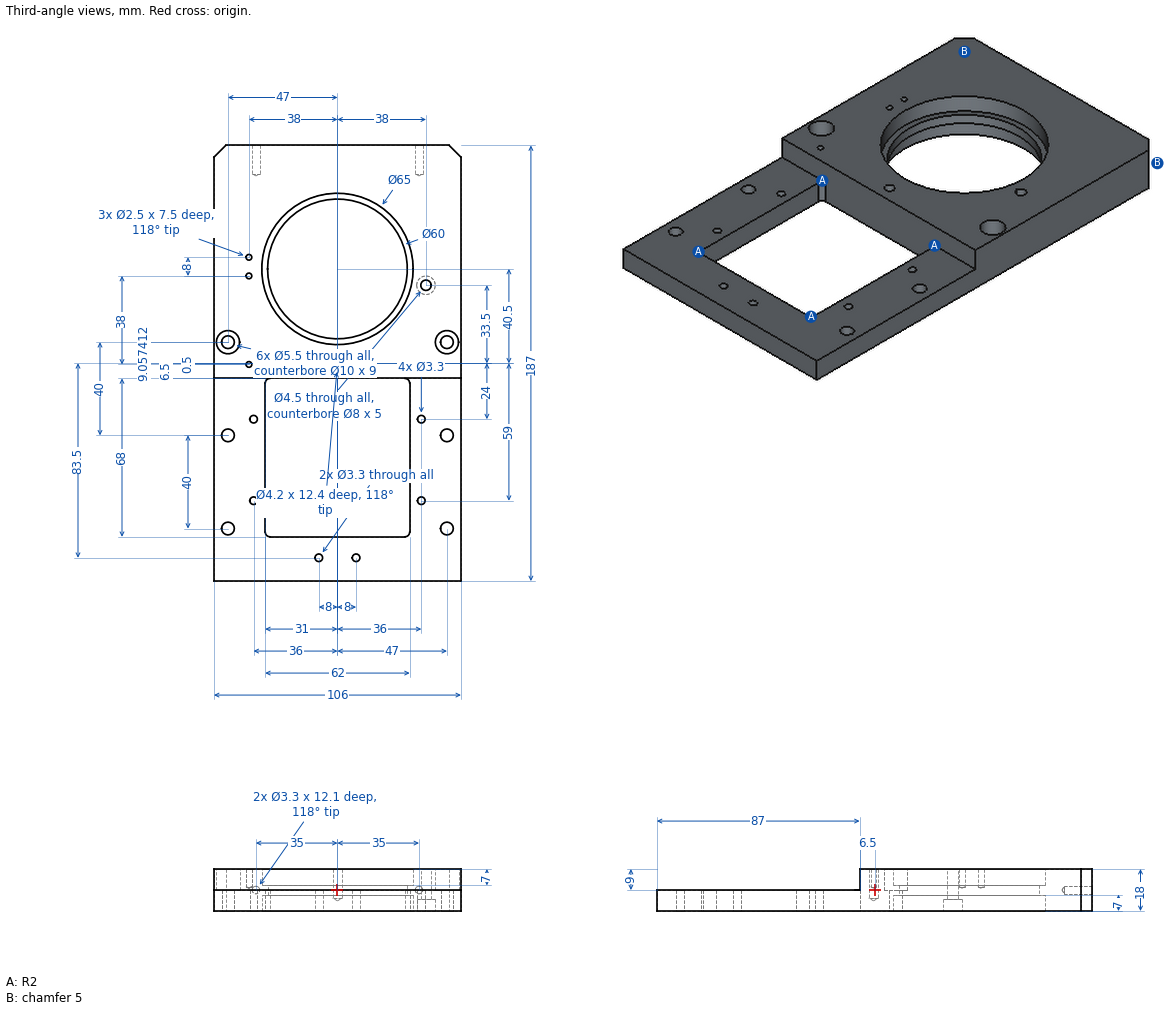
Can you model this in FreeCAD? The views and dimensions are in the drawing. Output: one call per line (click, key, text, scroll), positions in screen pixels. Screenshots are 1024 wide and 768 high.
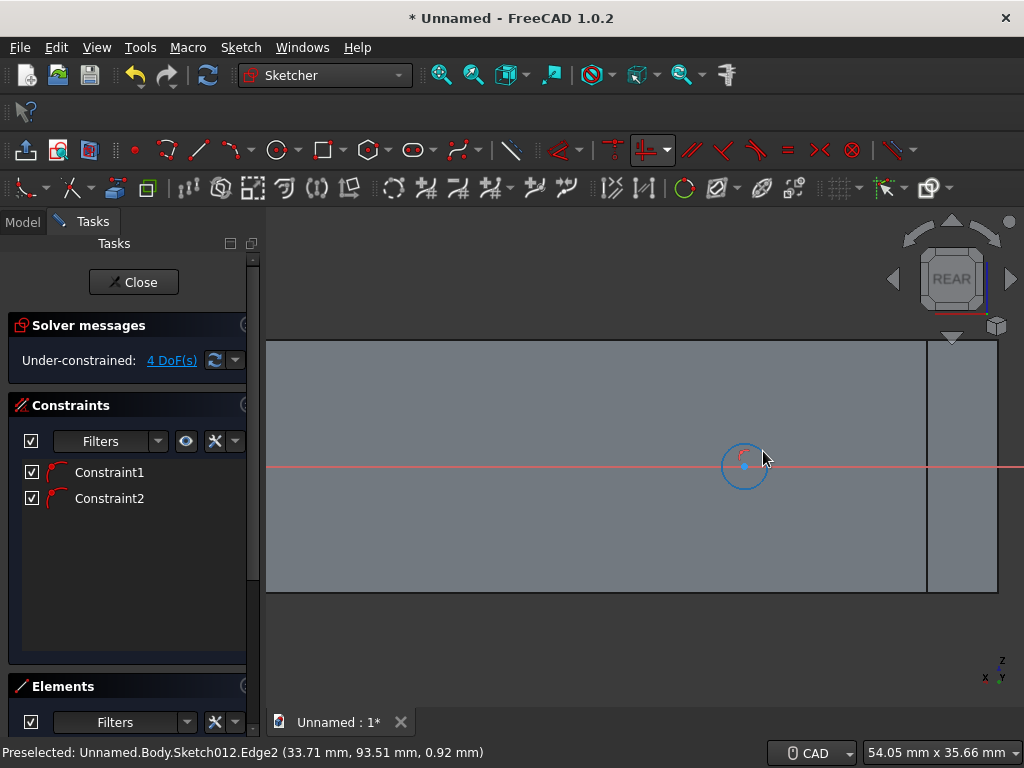
click(761, 450)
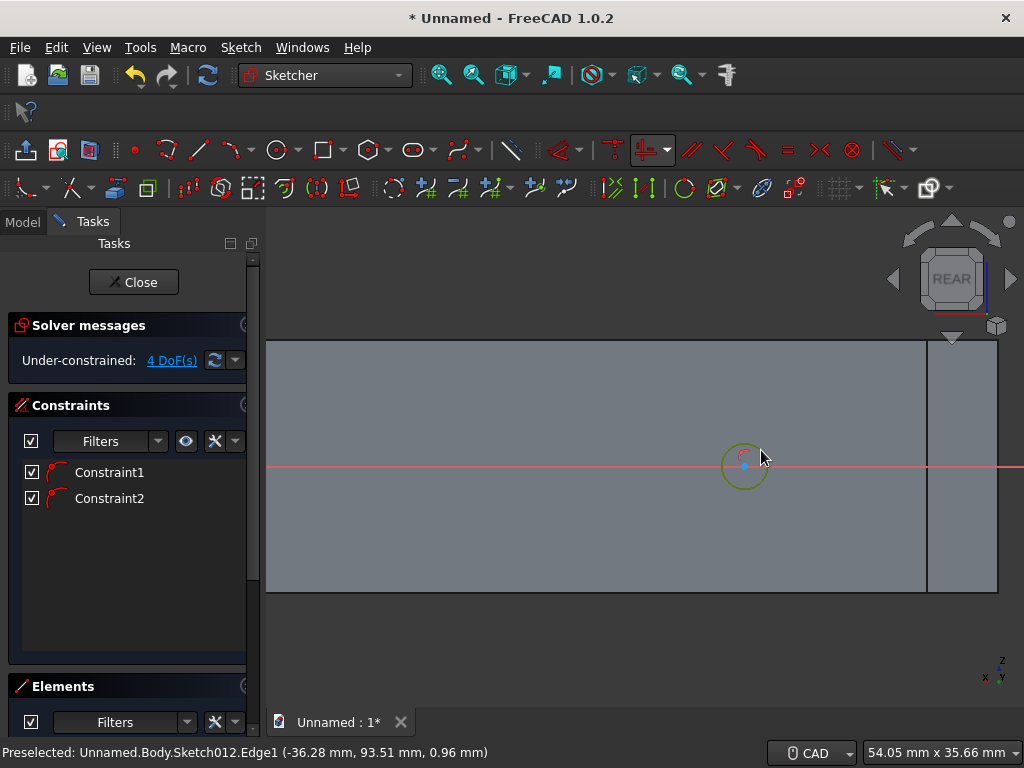
scroll(764, 451, down, 5)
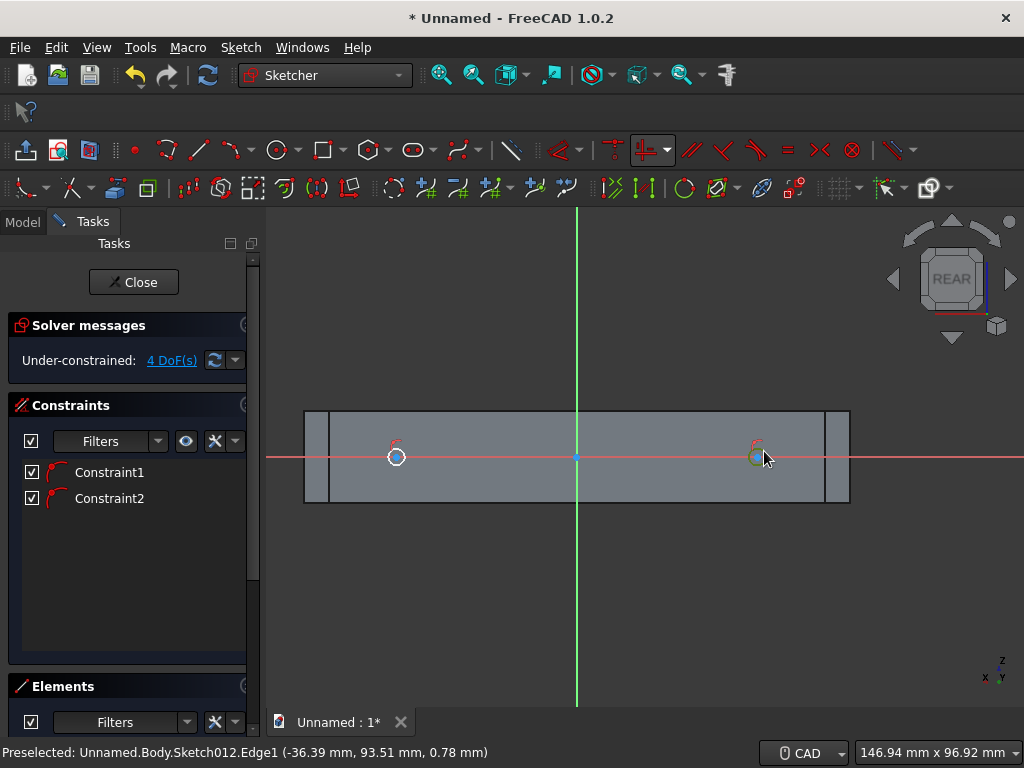
scroll(402, 451, up, 5)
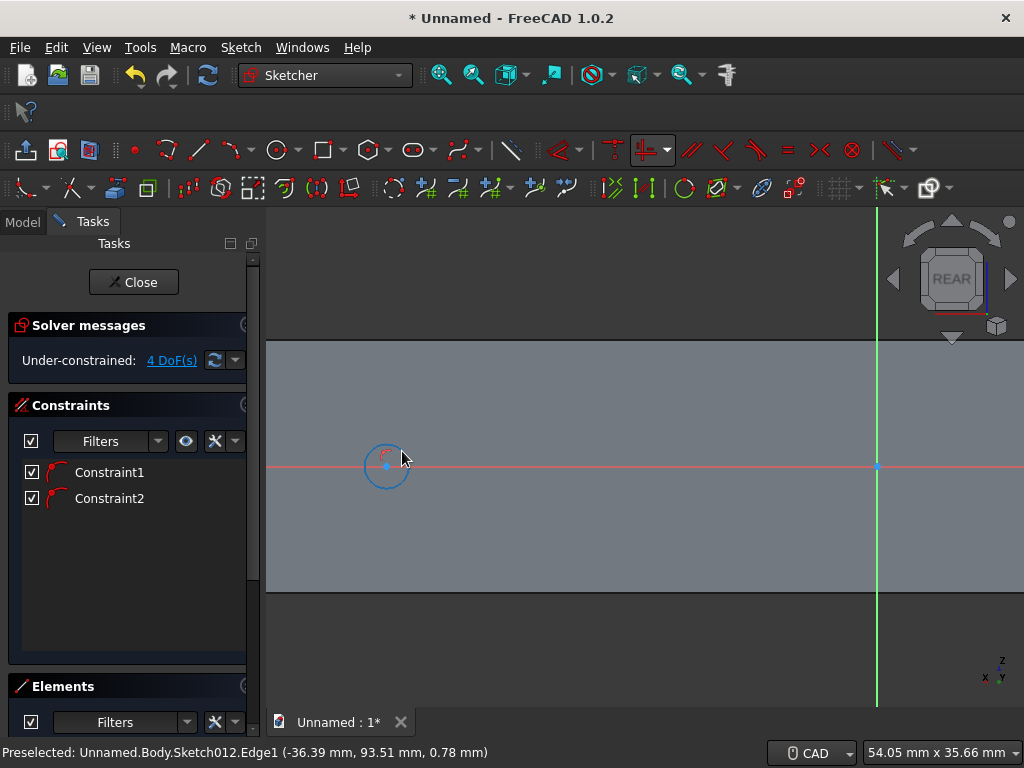
click(402, 451)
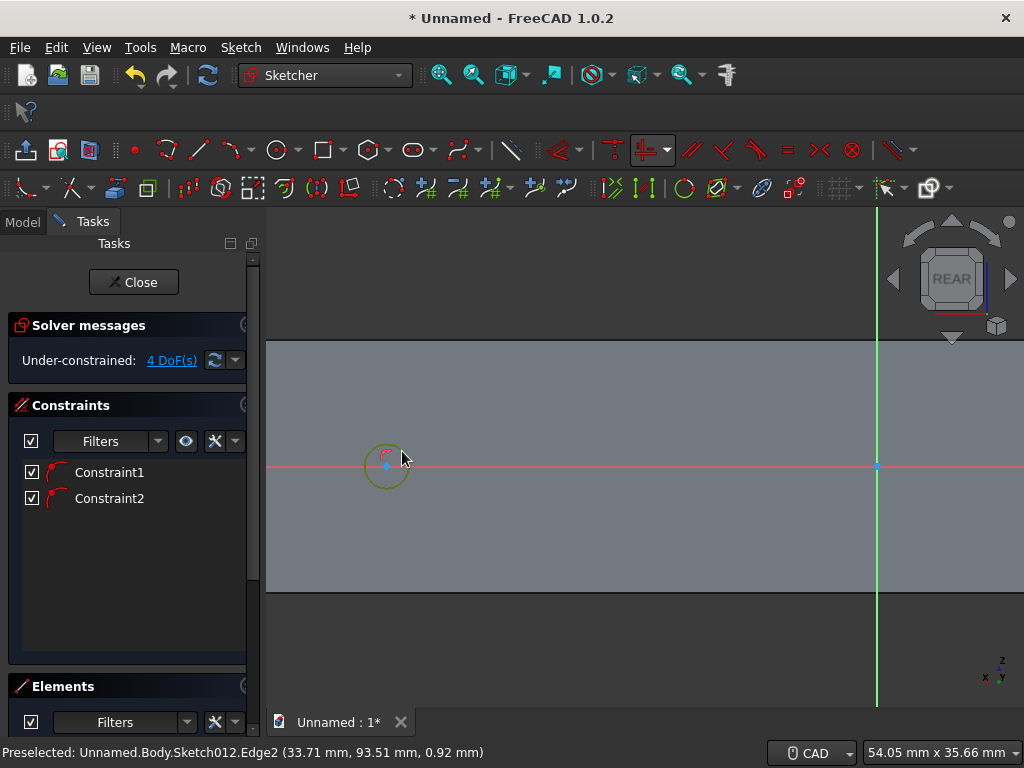
click(788, 150)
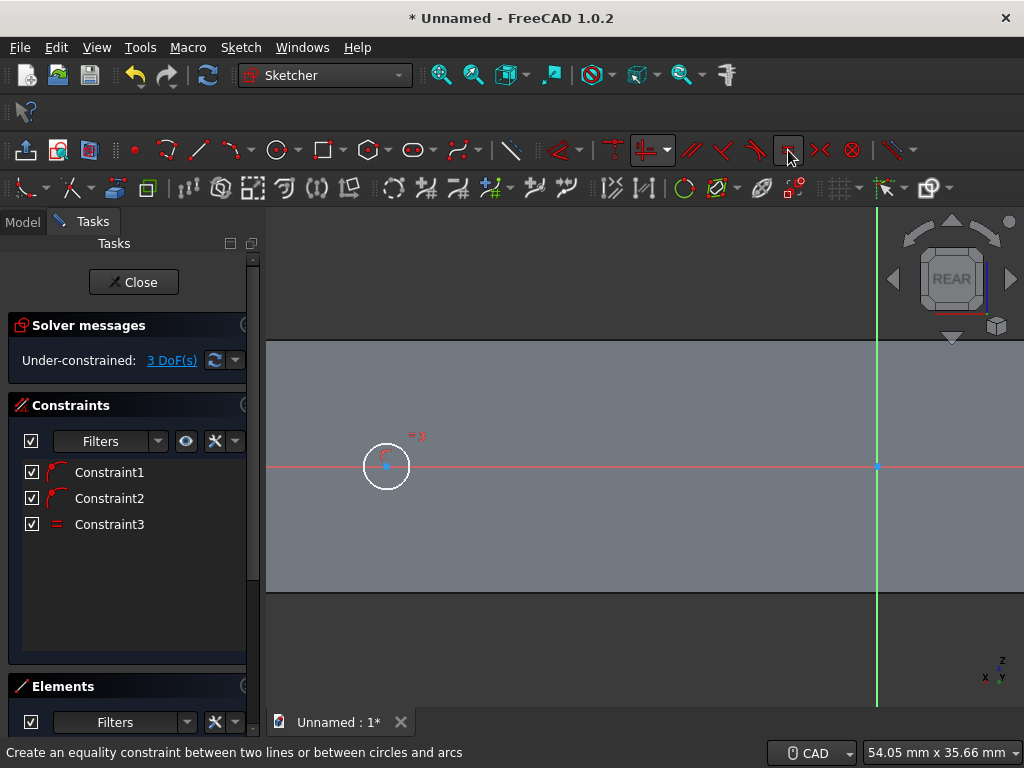
click(558, 150)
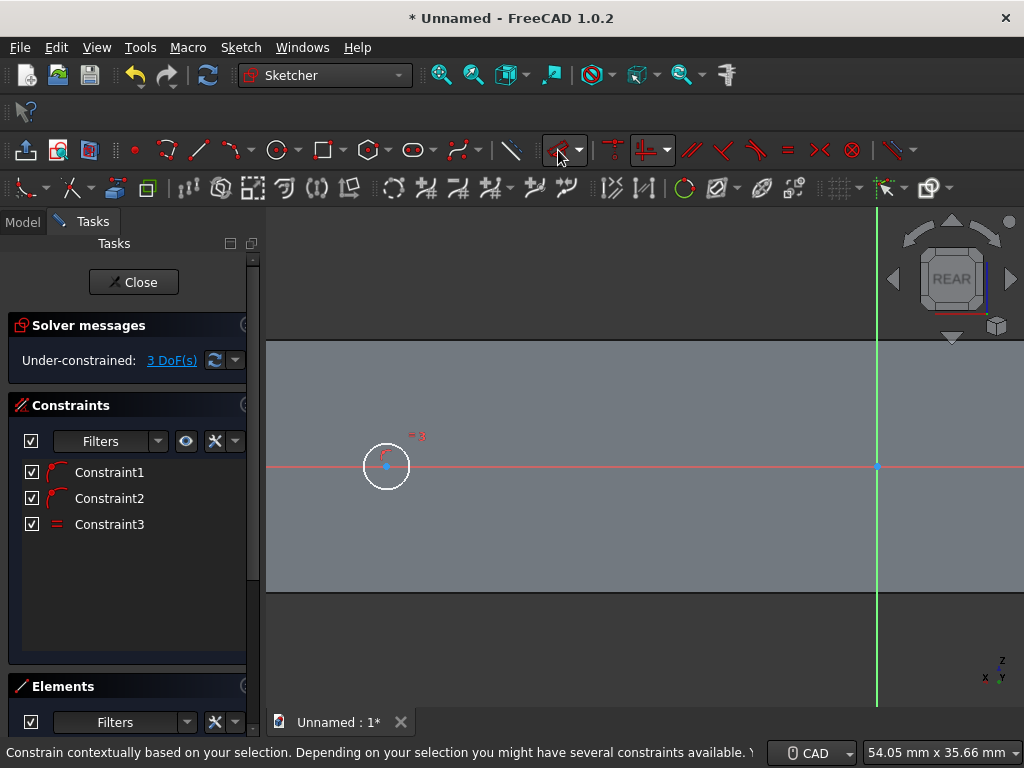
scroll(401, 451, down, 5)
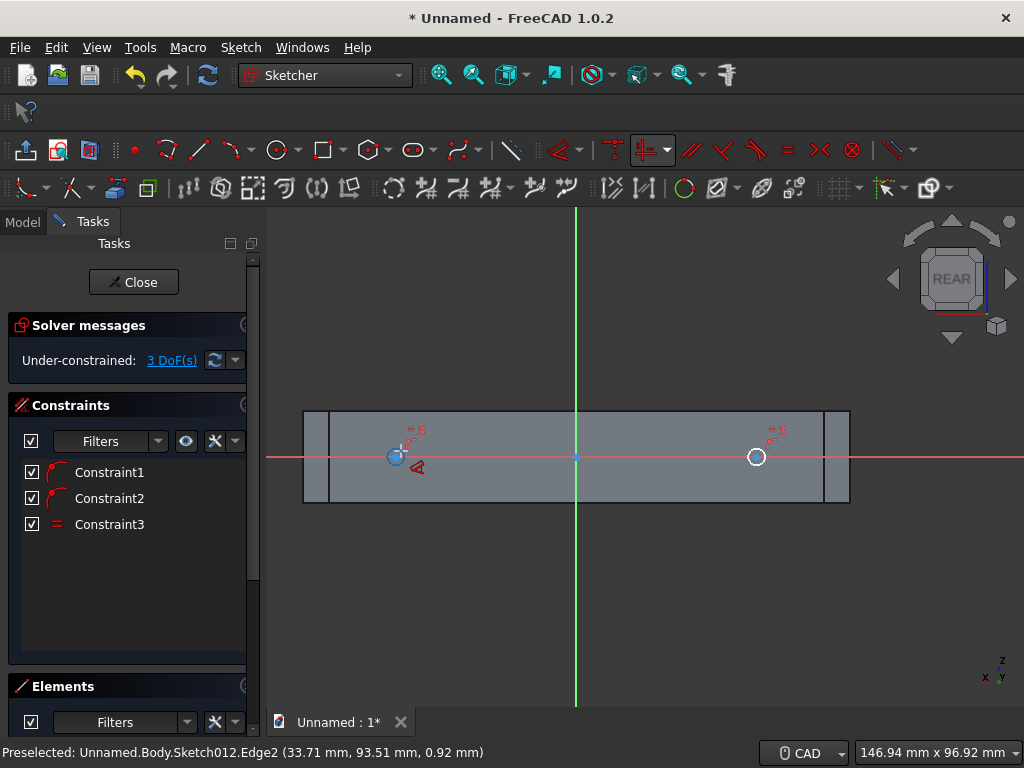
scroll(763, 451, up, 5)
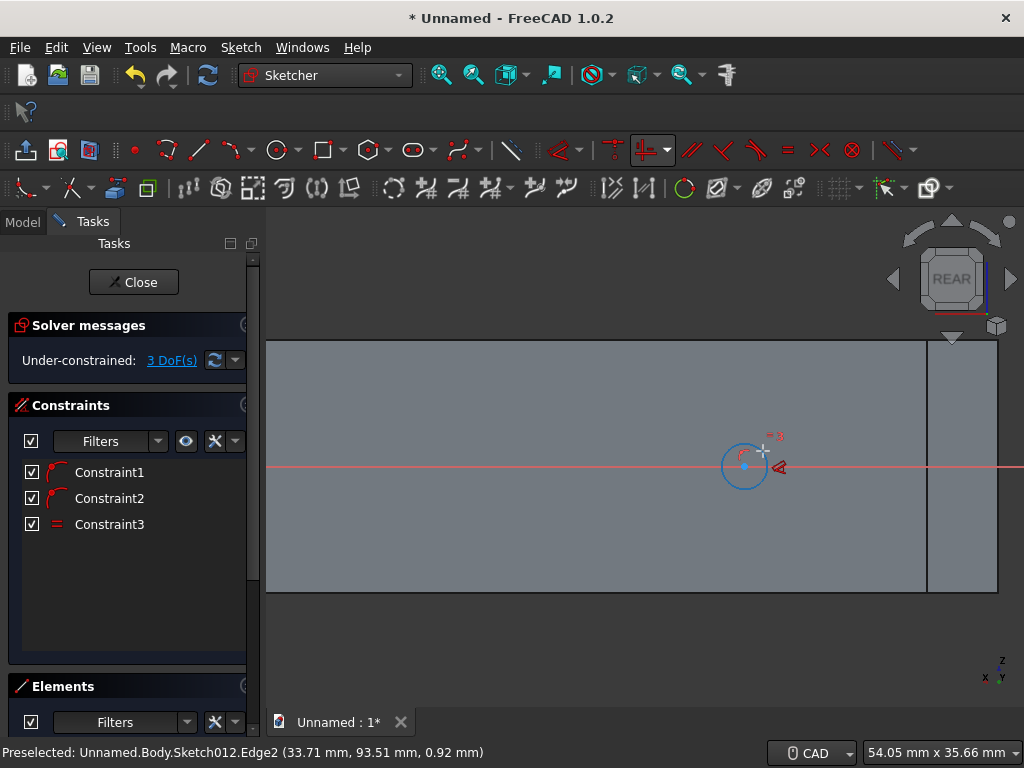
click(761, 450)
click(783, 427)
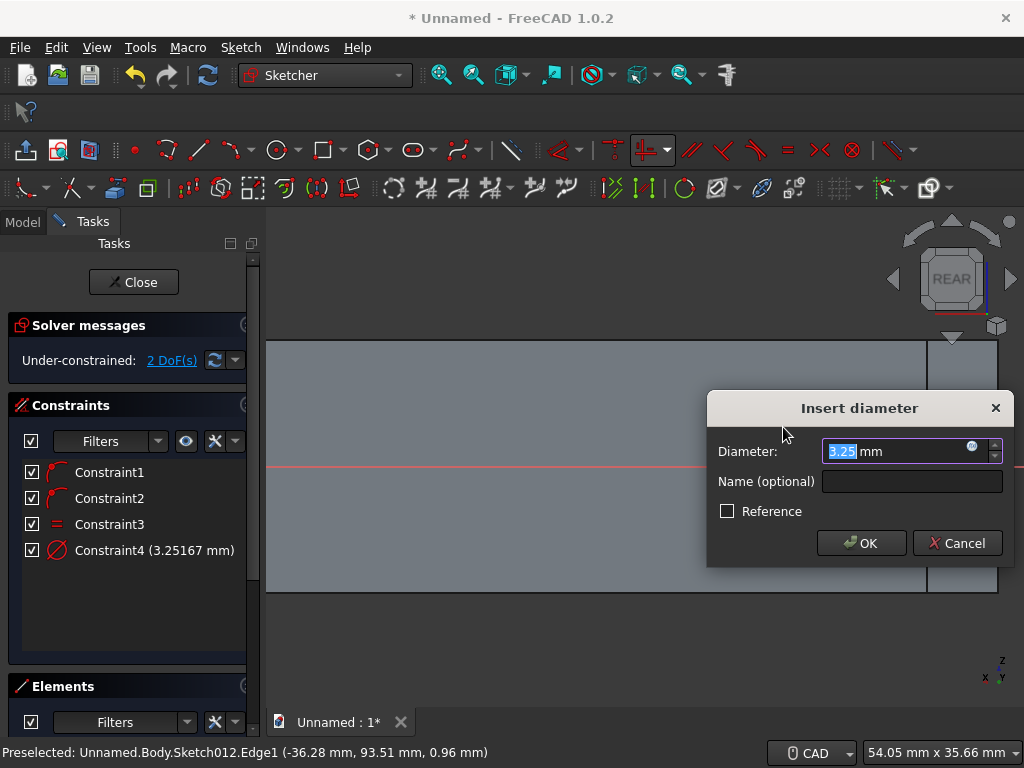
text(3.3)
key(Return)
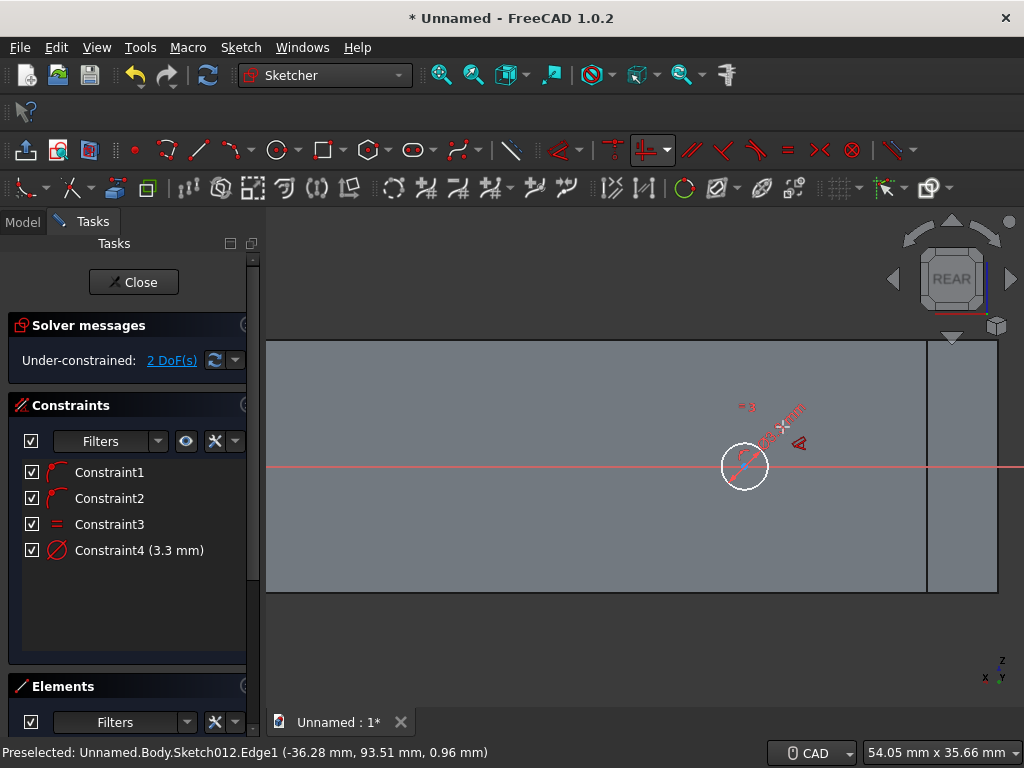
click(745, 467)
click(519, 501)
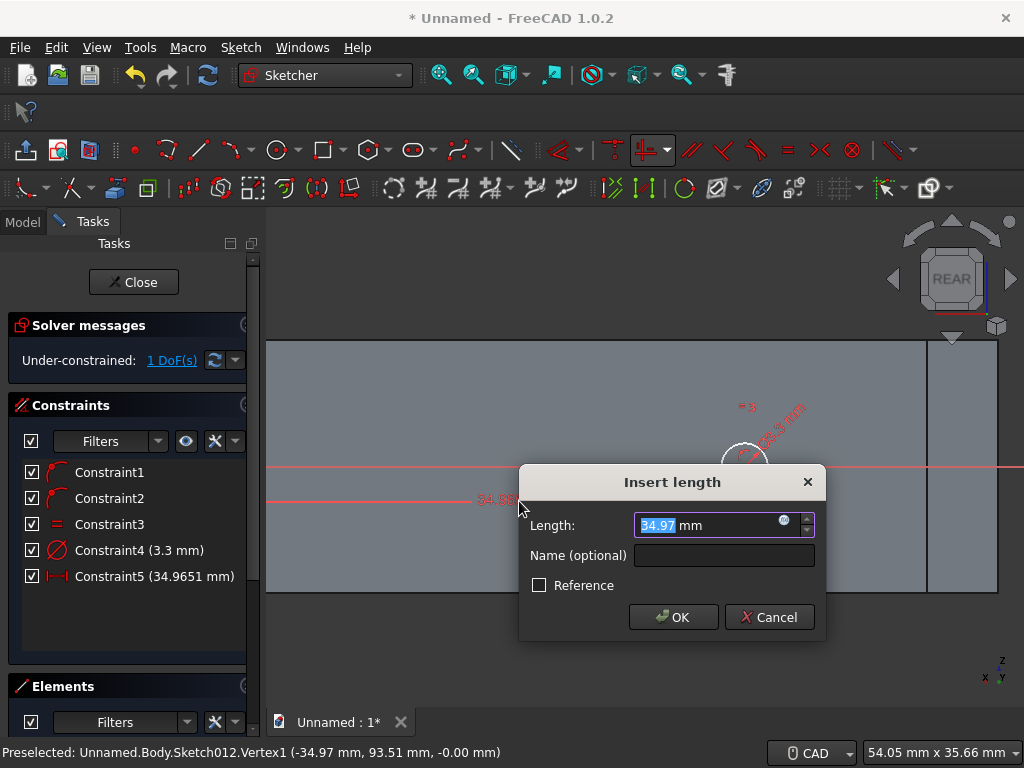
text(35)
key(Return)